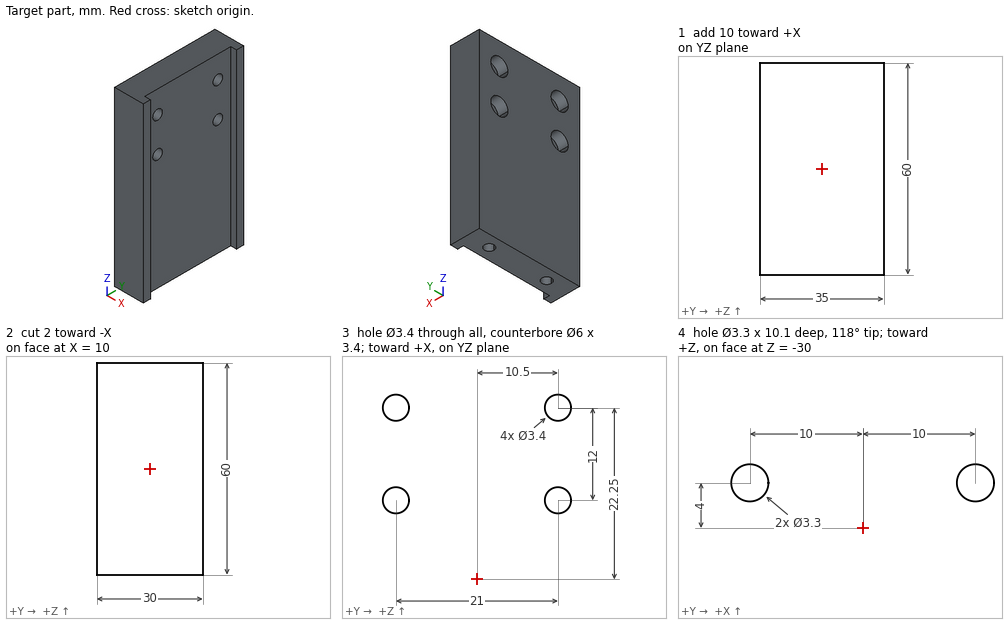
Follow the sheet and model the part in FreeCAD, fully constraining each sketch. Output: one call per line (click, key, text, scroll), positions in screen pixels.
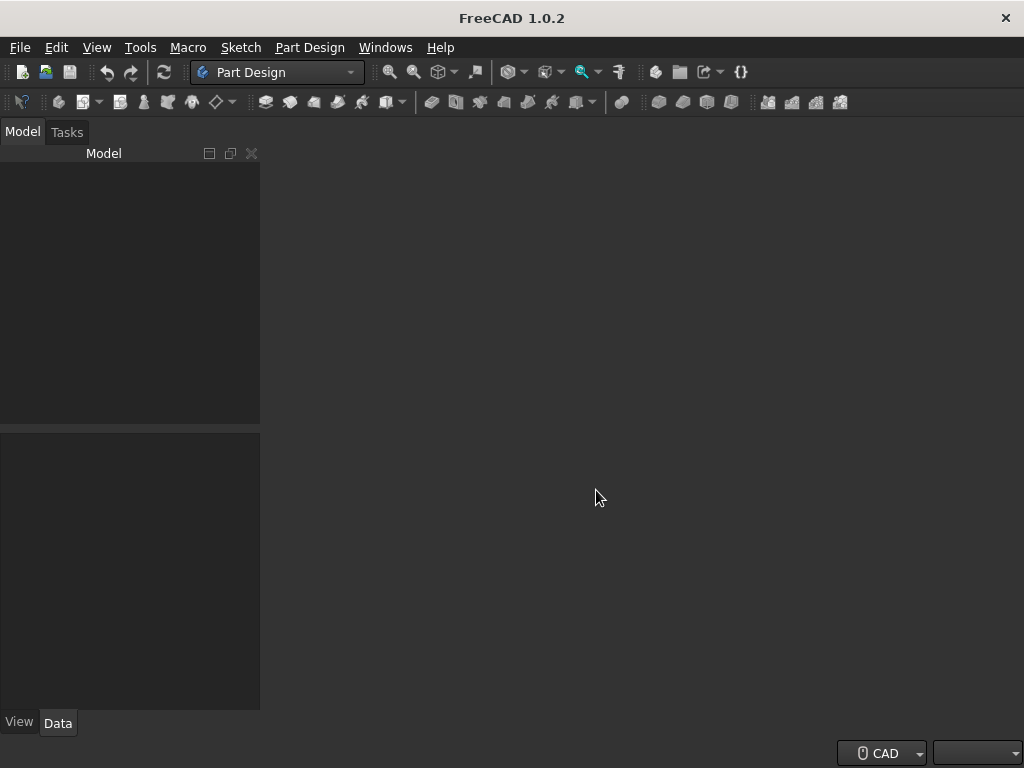
click(22, 72)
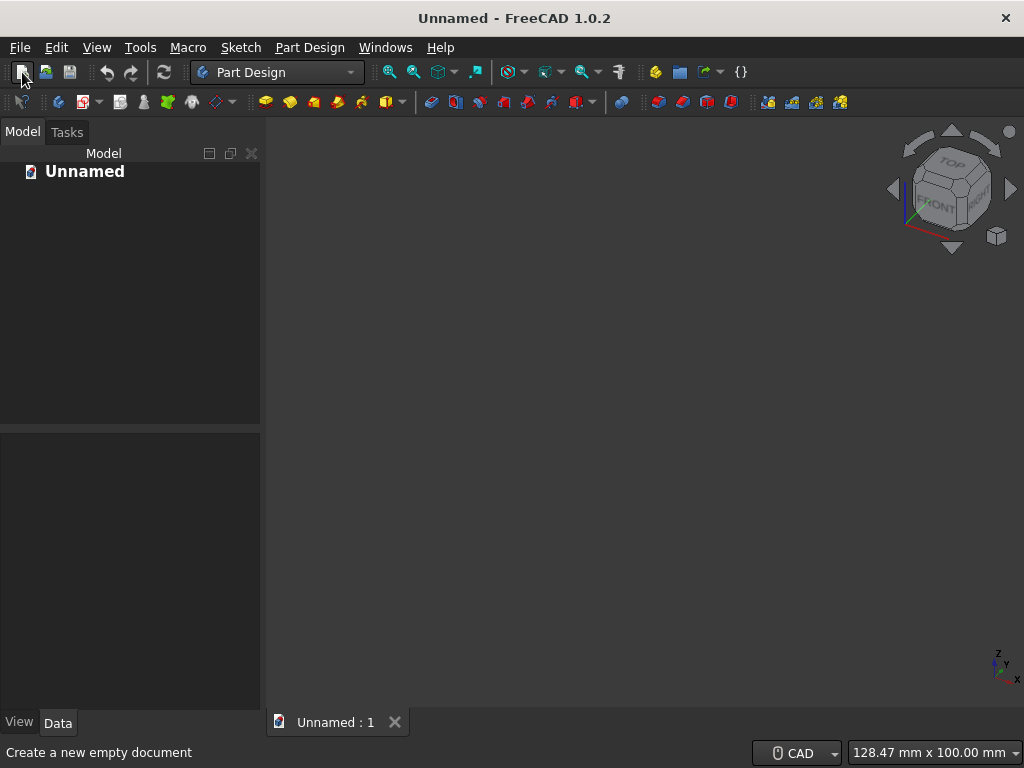
click(84, 102)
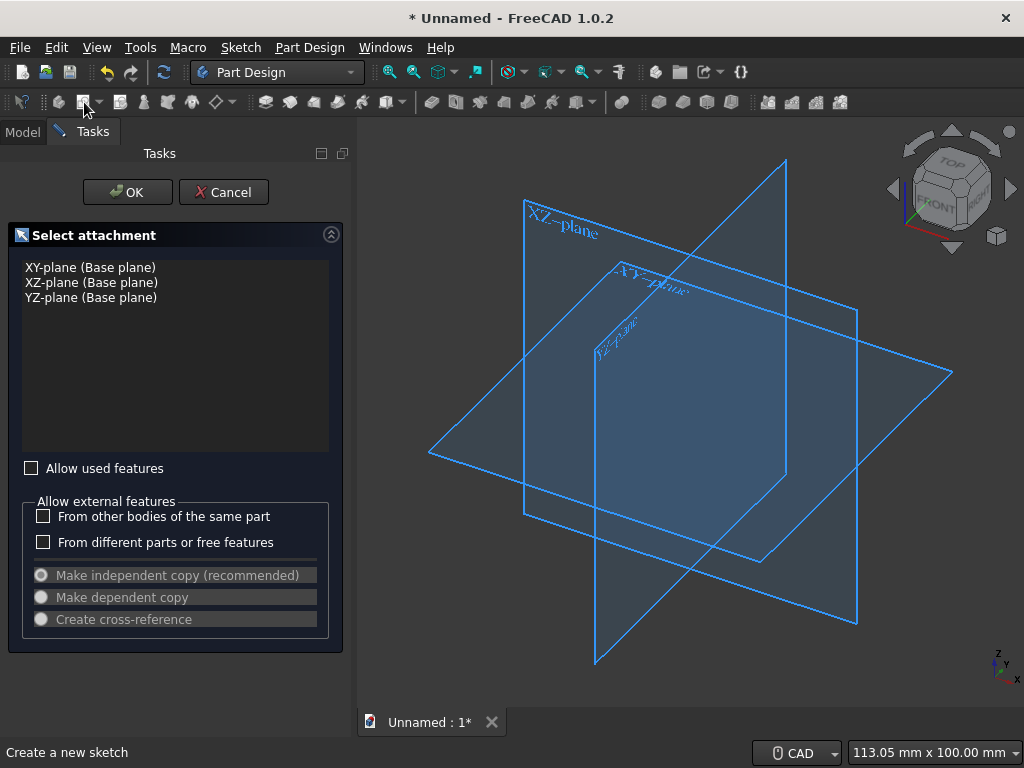
click(82, 298)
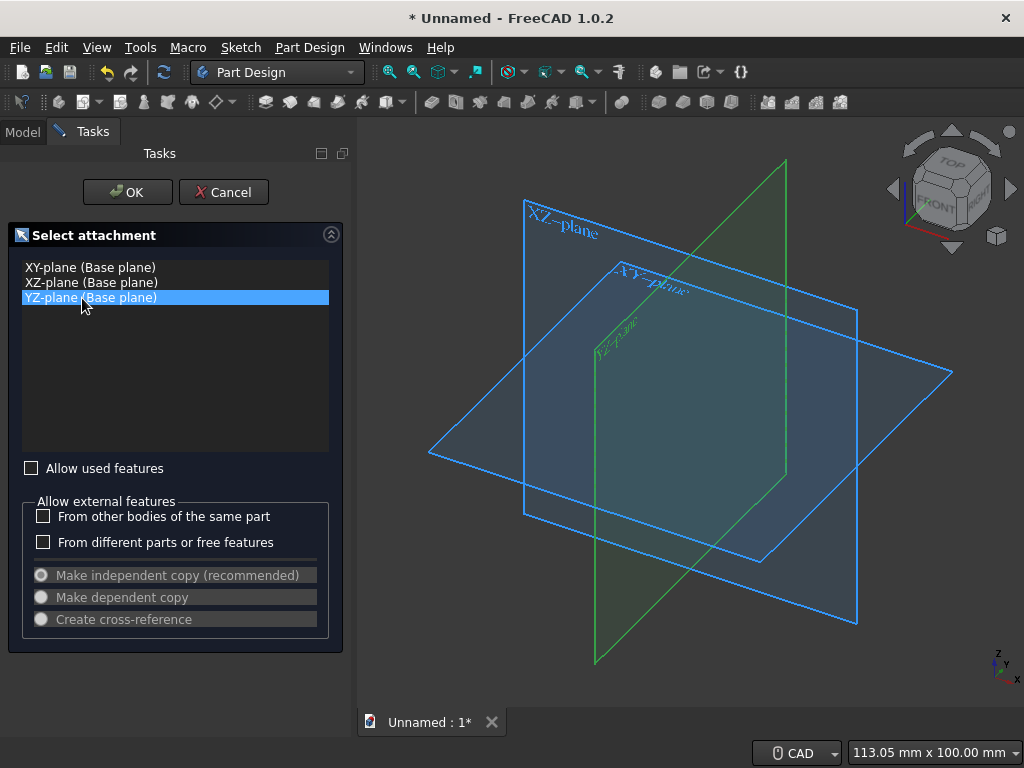
click(128, 192)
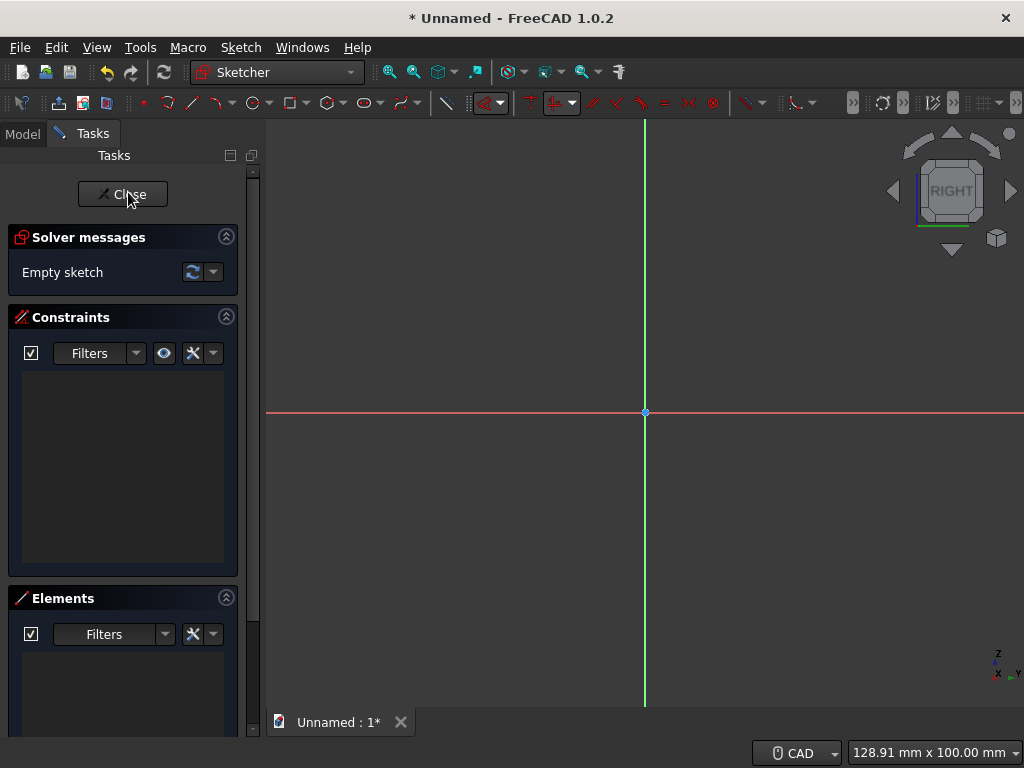
click(308, 104)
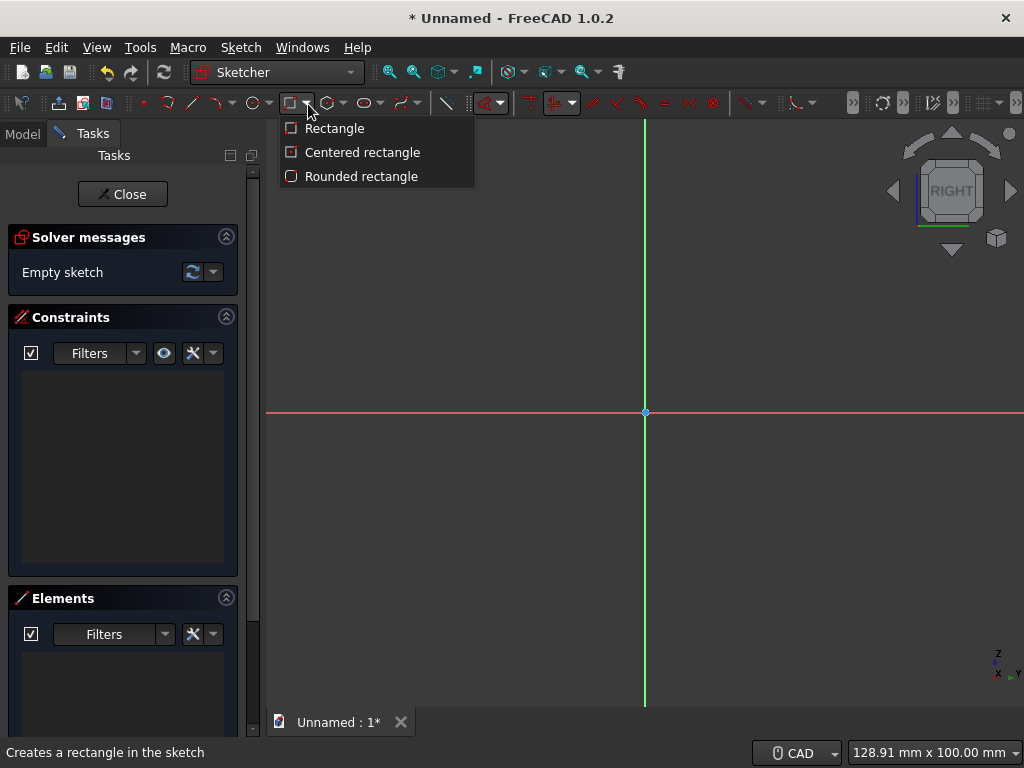
click(378, 152)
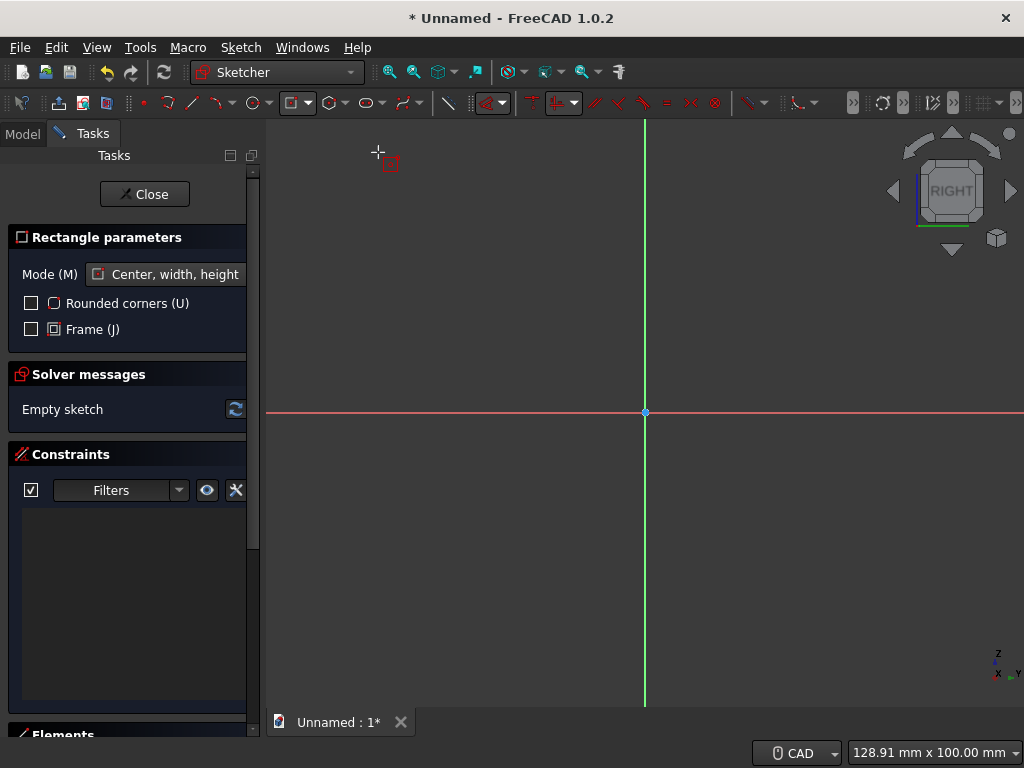
click(645, 413)
move(748, 237)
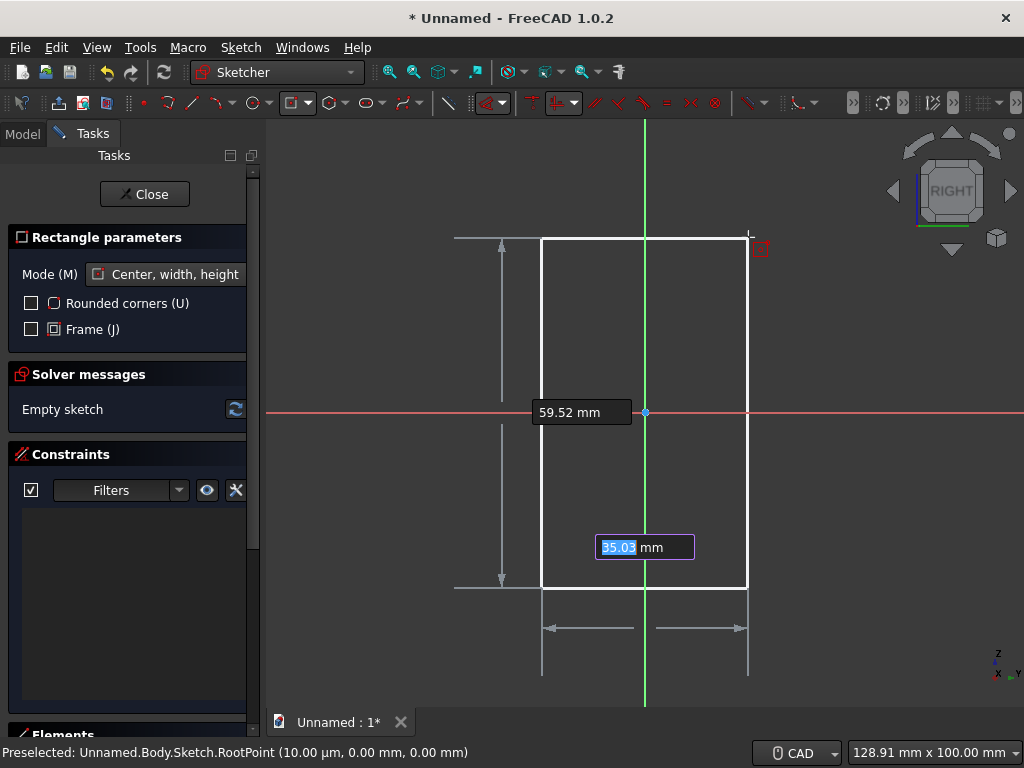
text(35)
key(Tab)
text(60)
key(Return)
key(Escape)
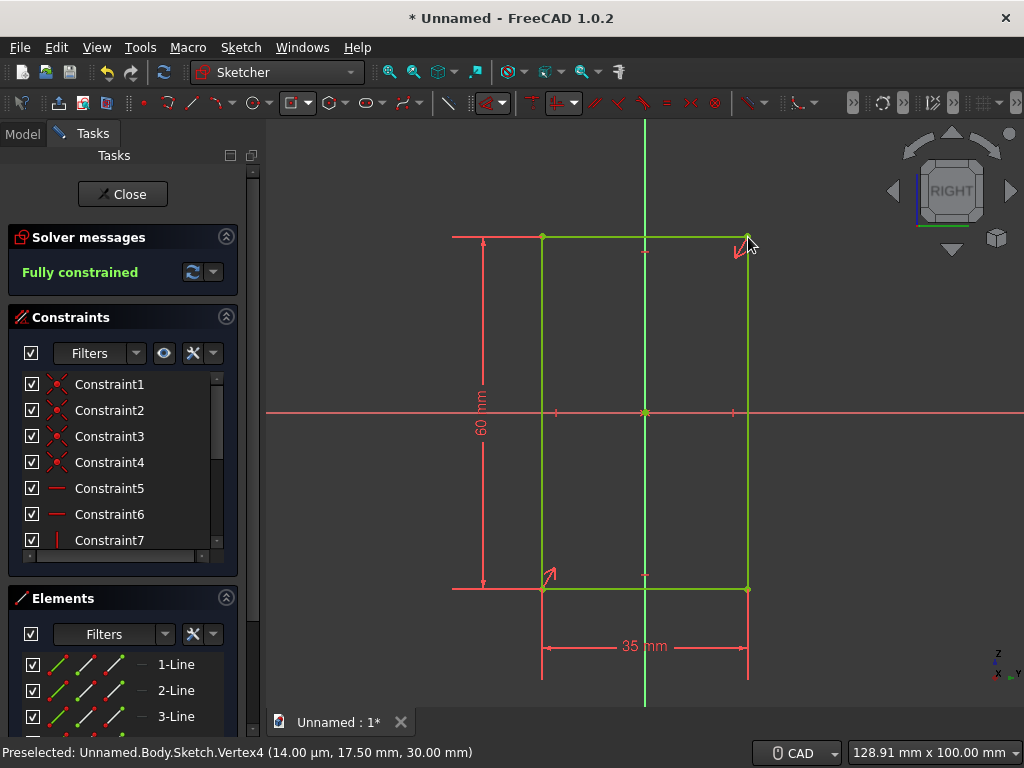
click(123, 194)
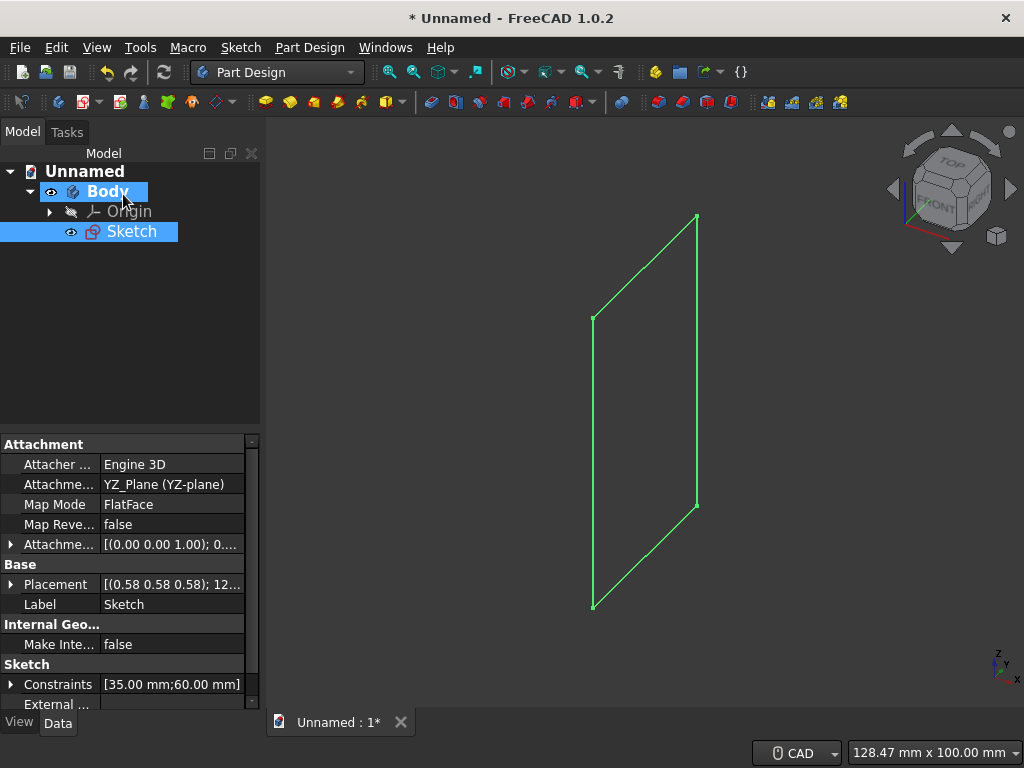
click(266, 102)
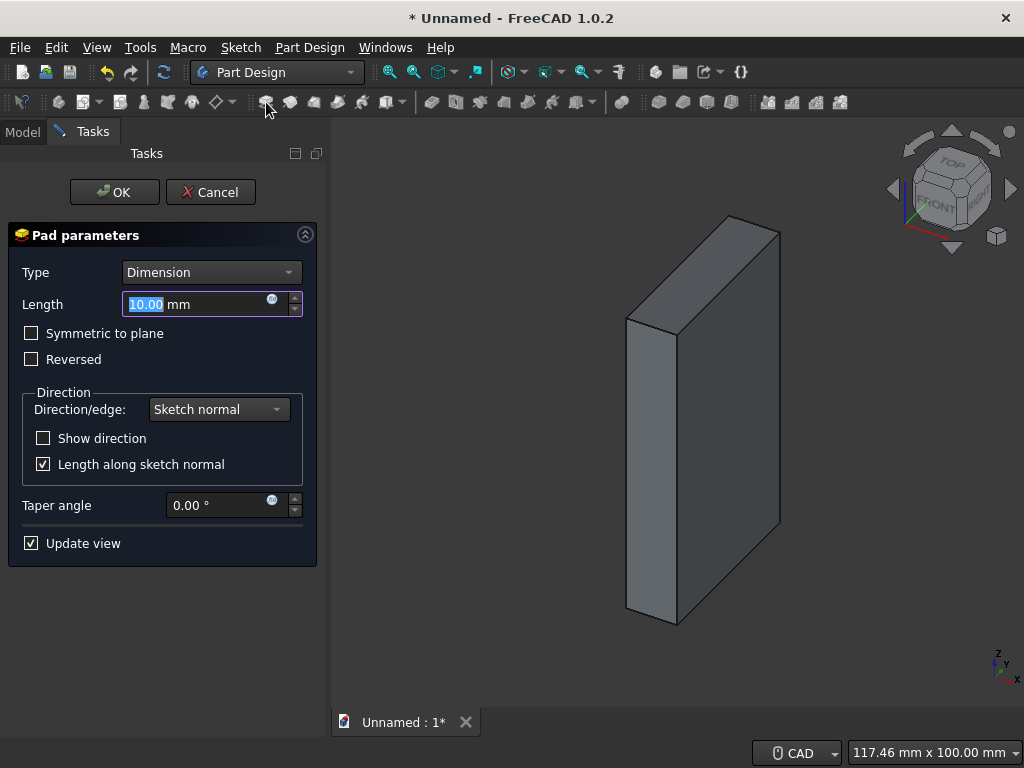
text(10)
key(Tab)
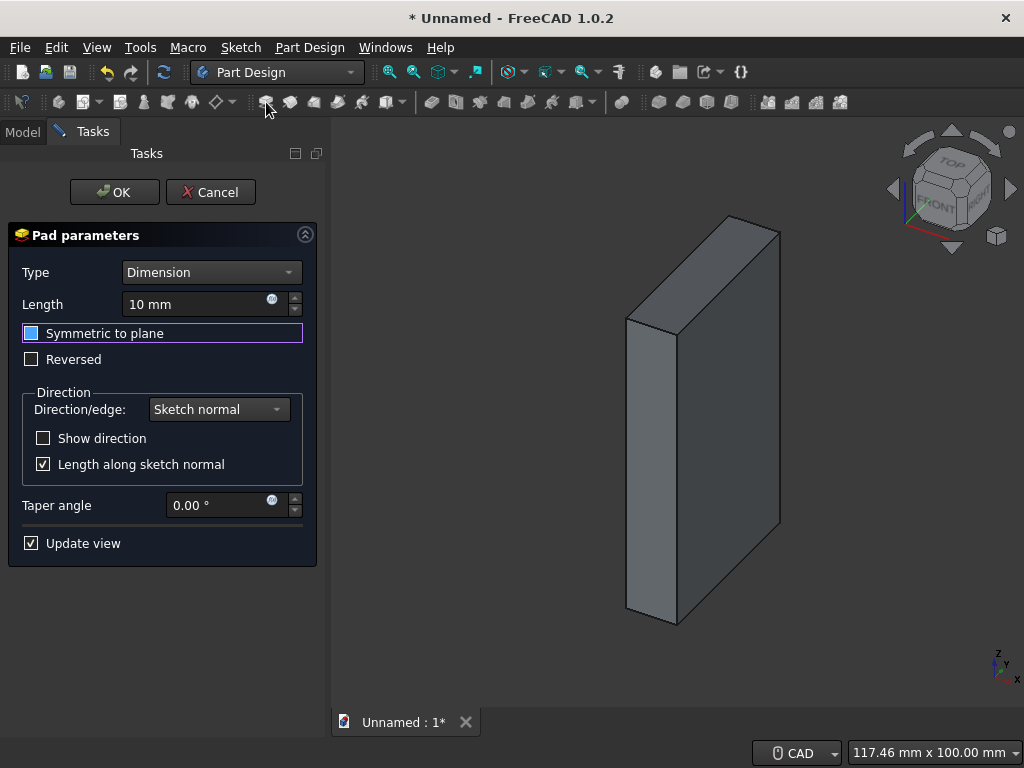
click(115, 192)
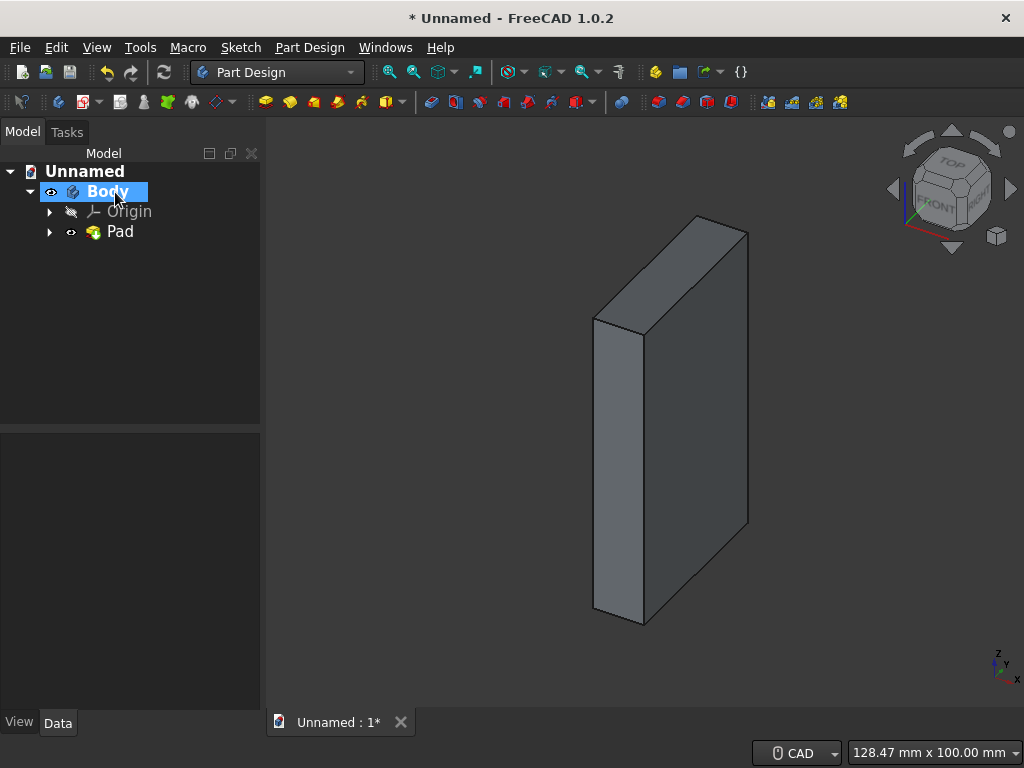
click(696, 469)